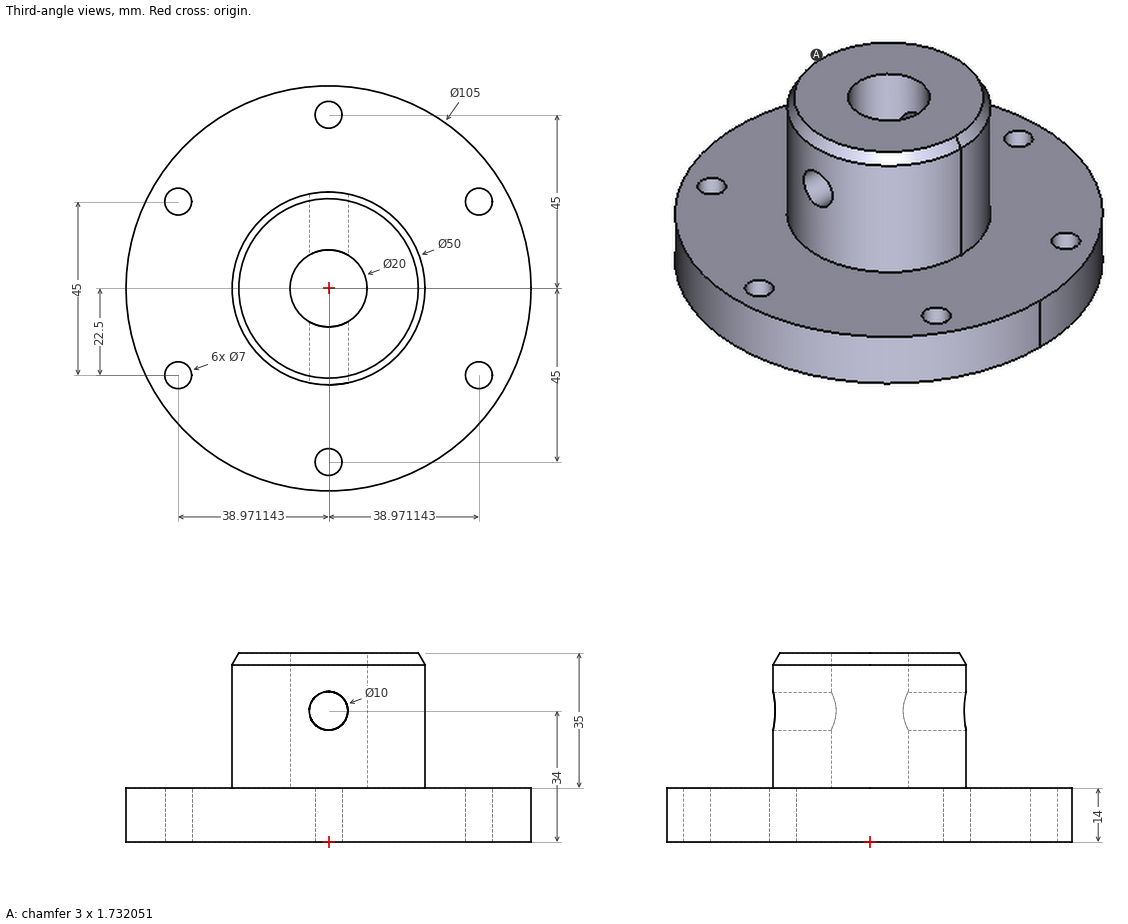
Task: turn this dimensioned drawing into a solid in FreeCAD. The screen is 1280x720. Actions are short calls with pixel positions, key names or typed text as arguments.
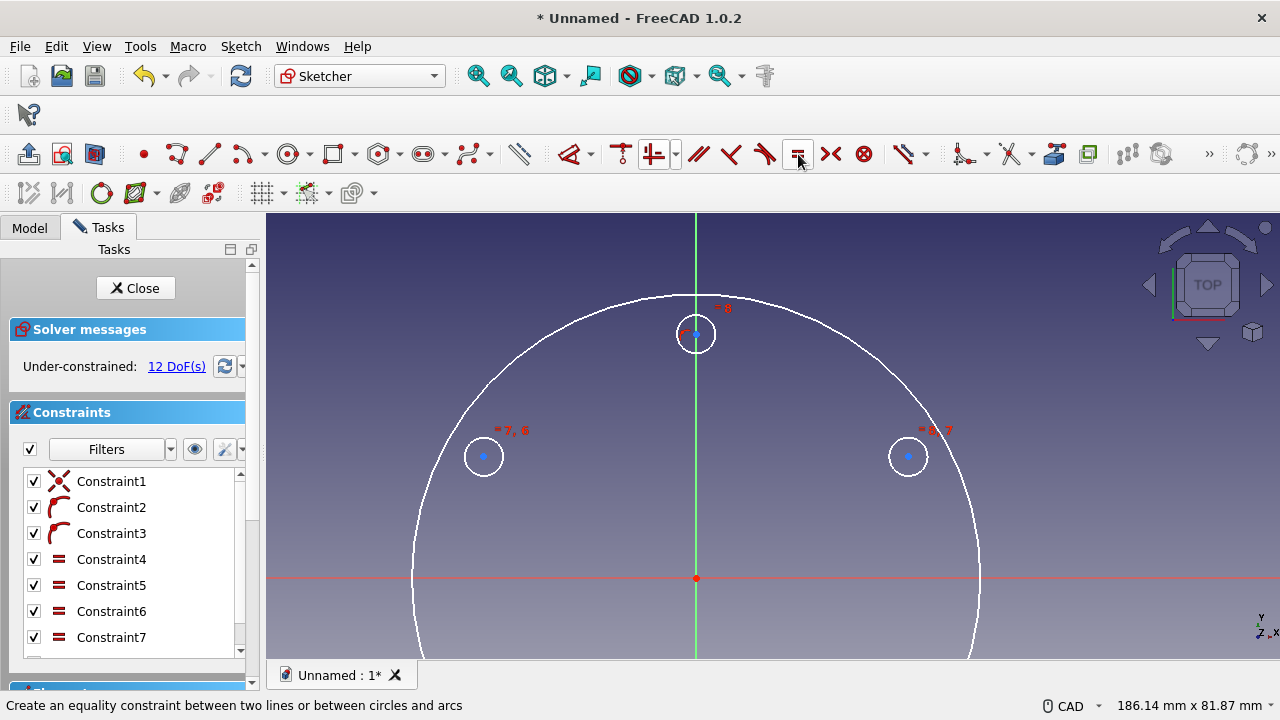
scroll(711, 320, down, 4)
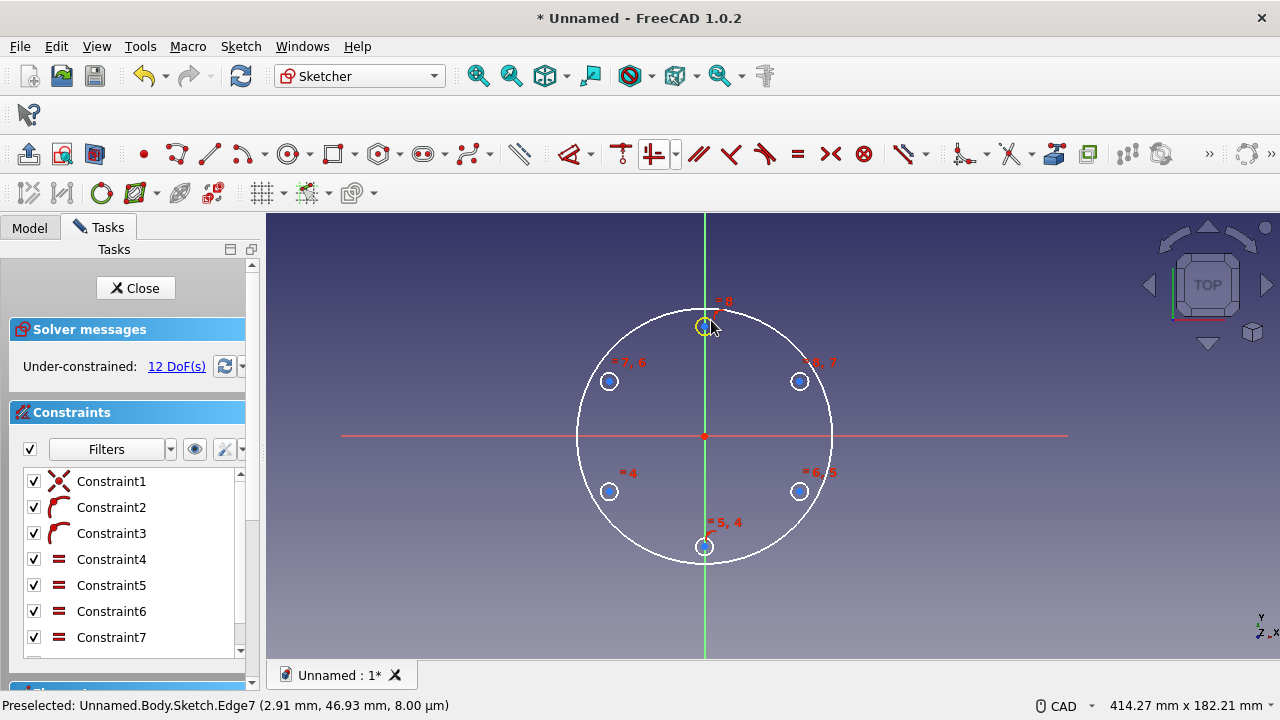
click(609, 492)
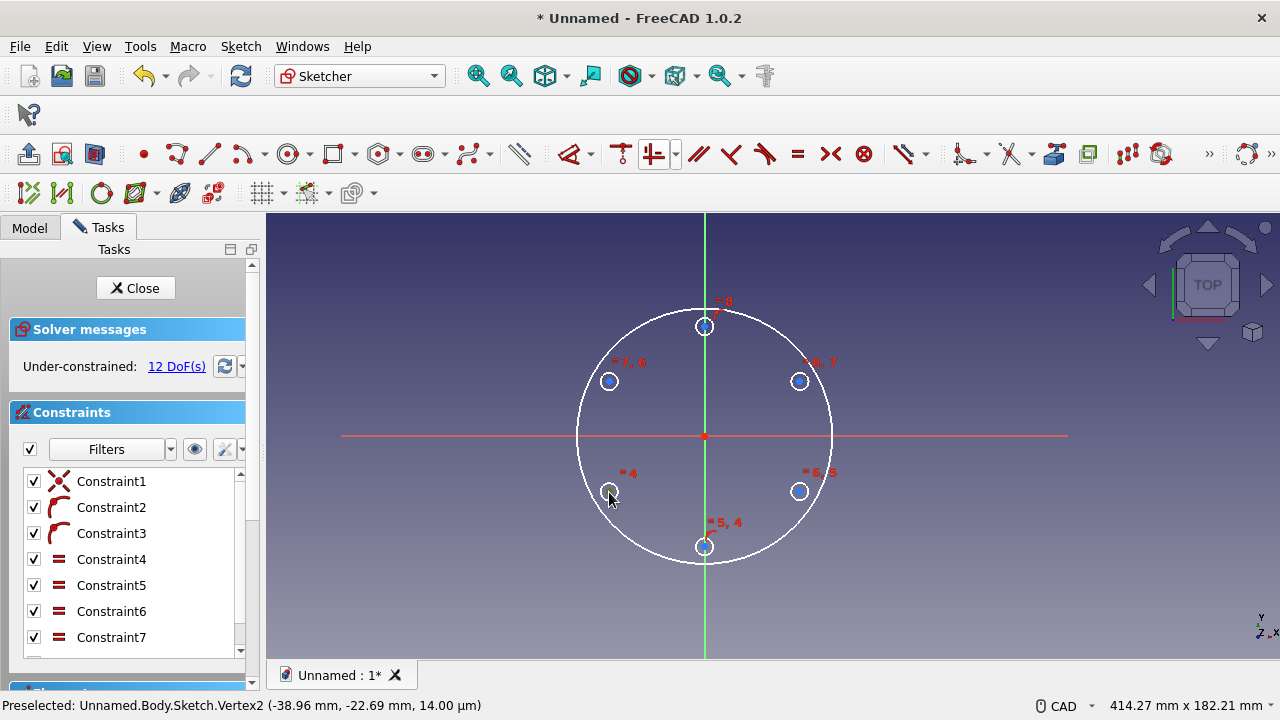
click(800, 492)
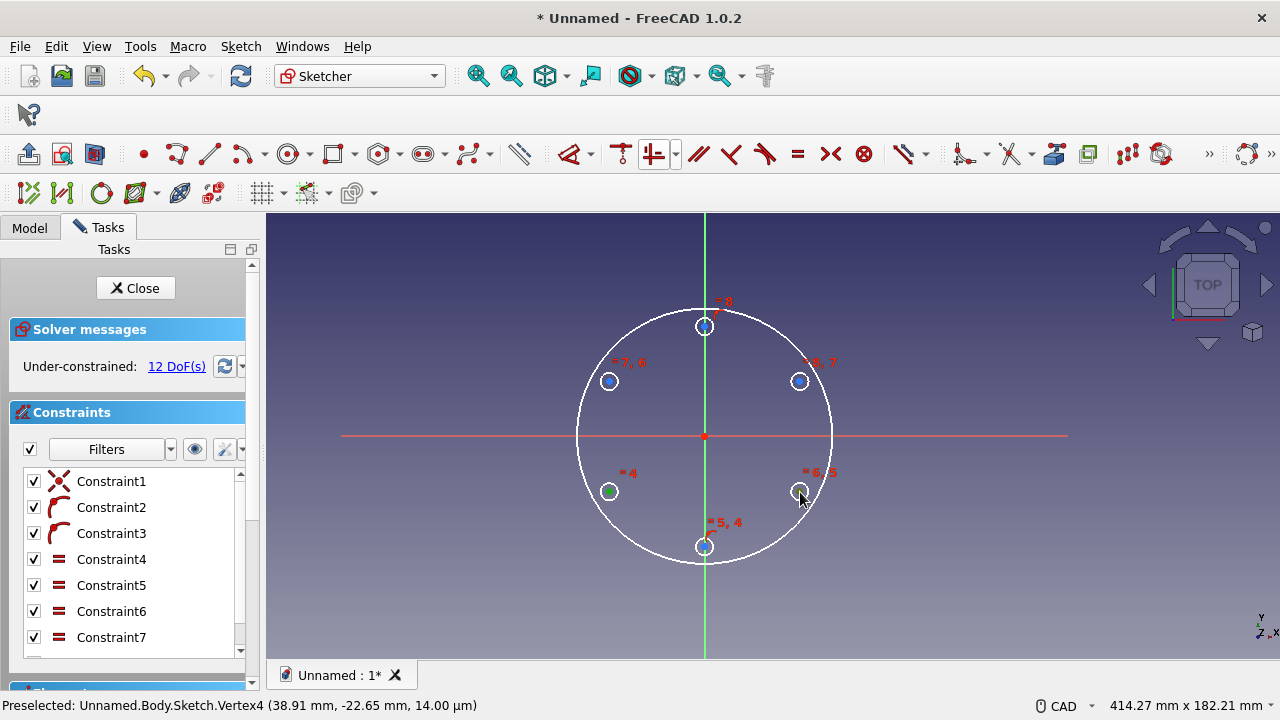
click(676, 154)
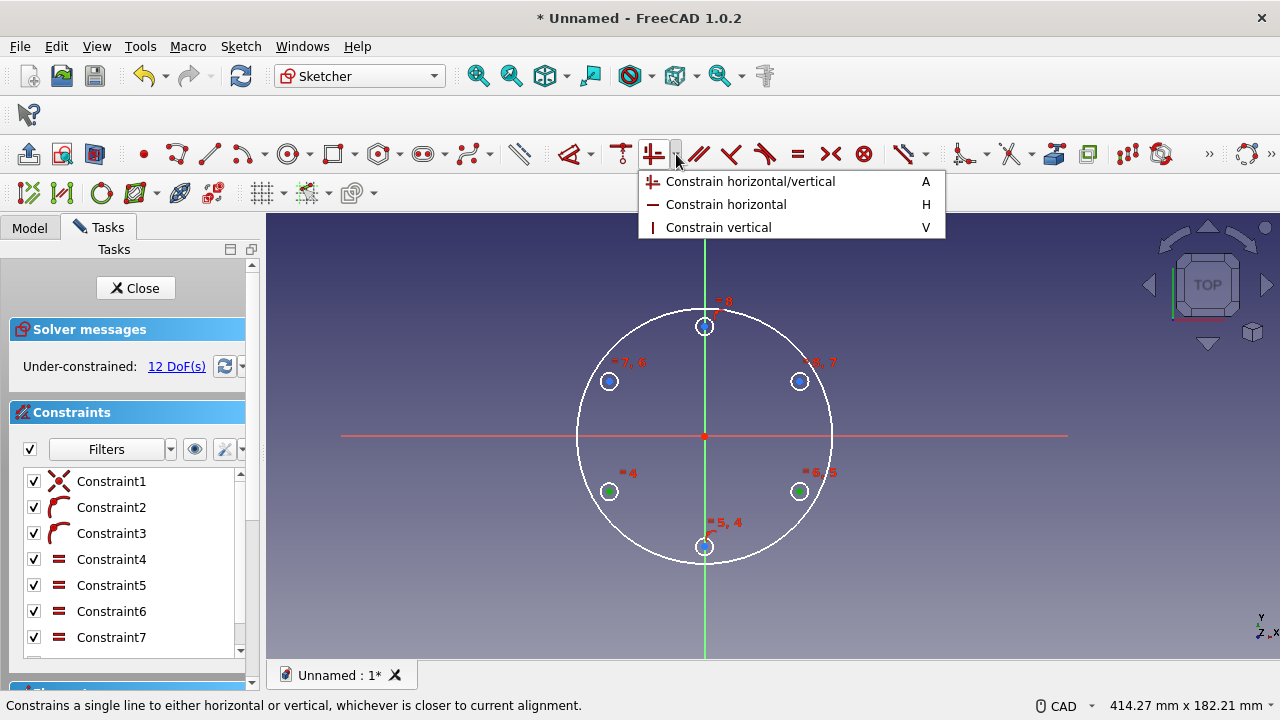
click(792, 204)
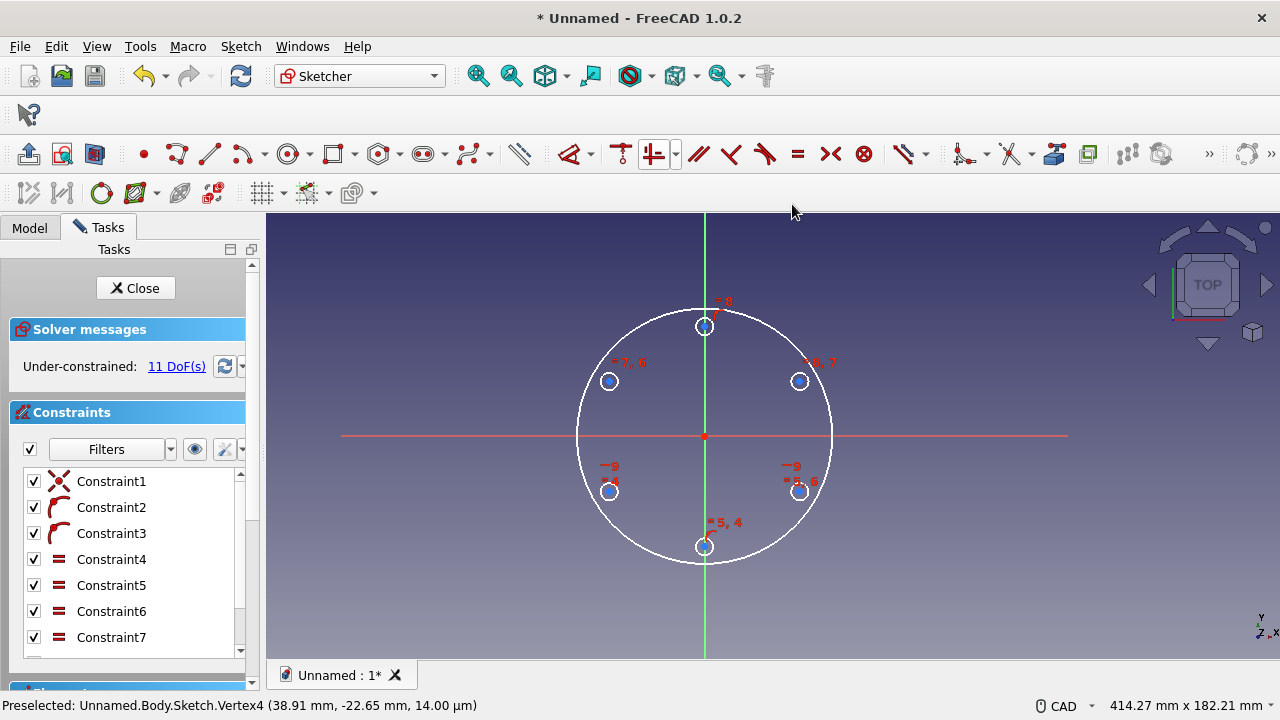
click(609, 492)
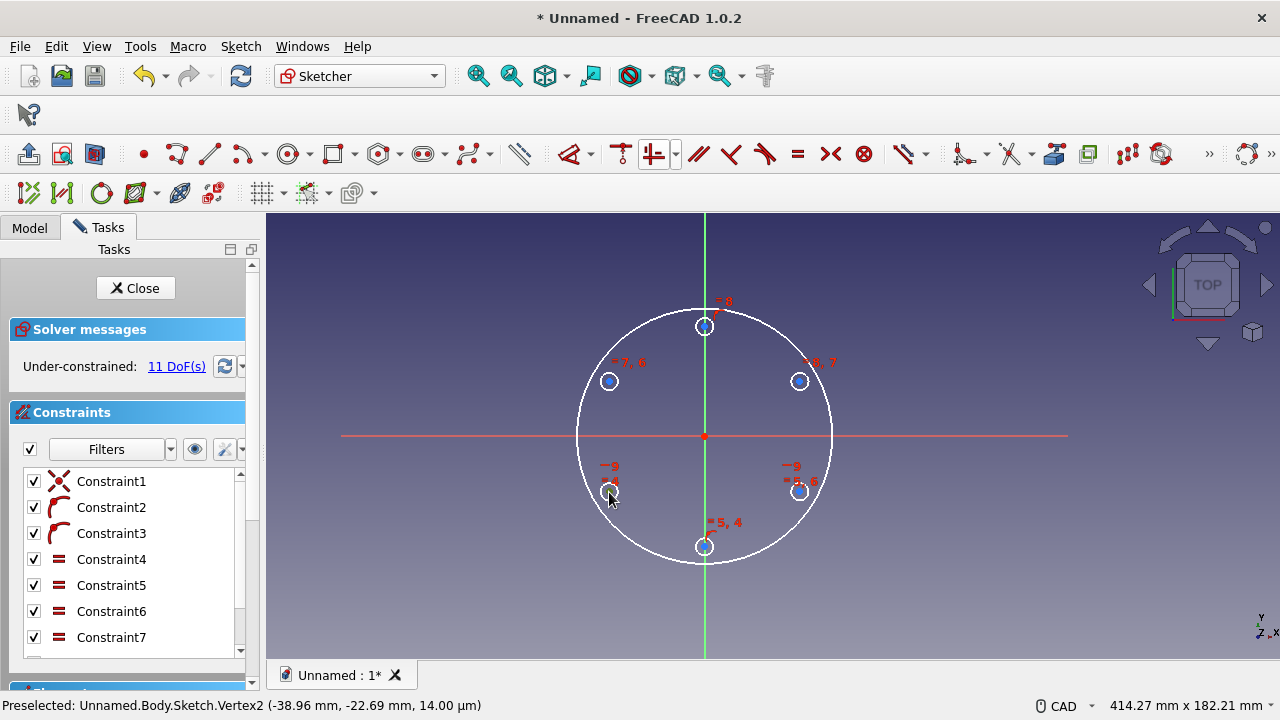
click(609, 382)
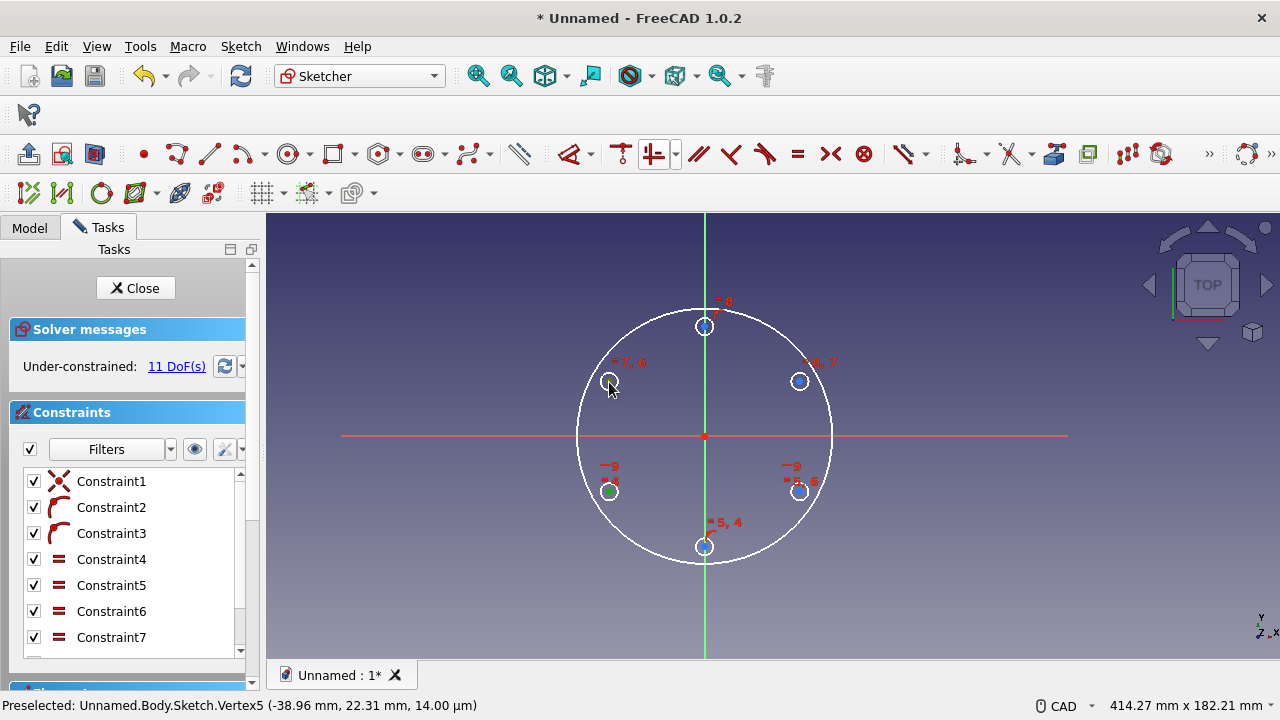
click(676, 154)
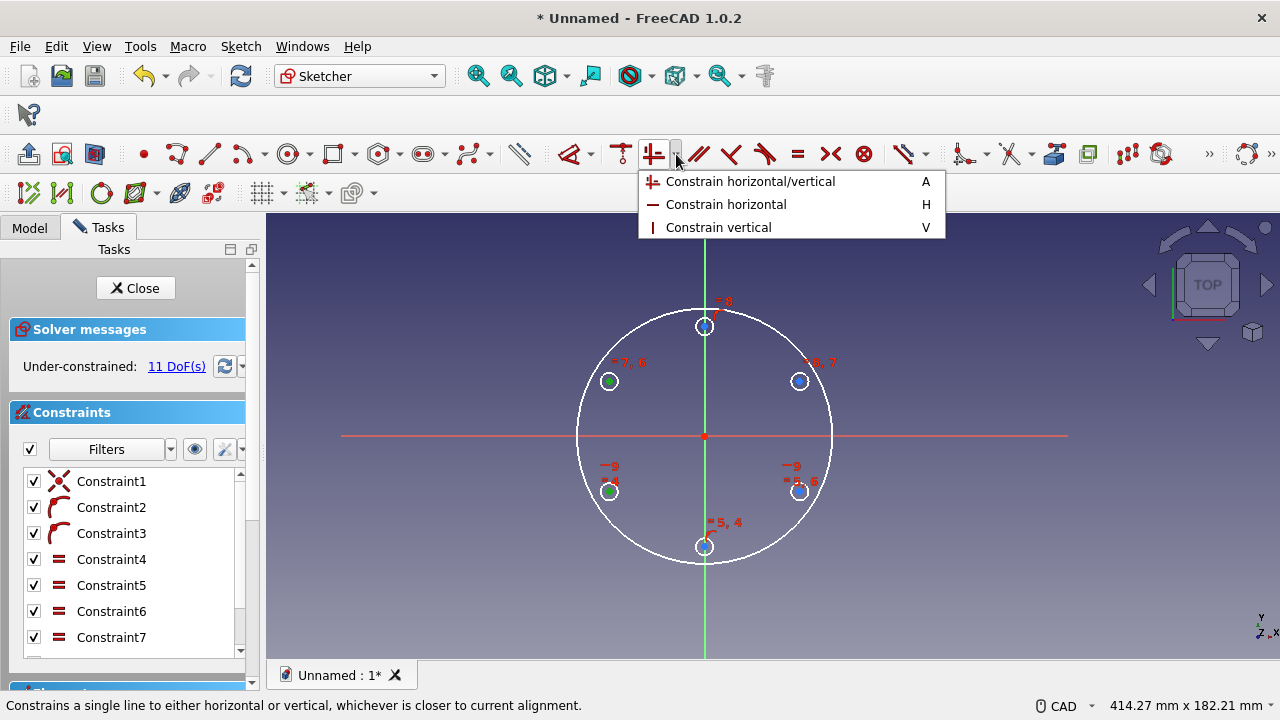
click(792, 228)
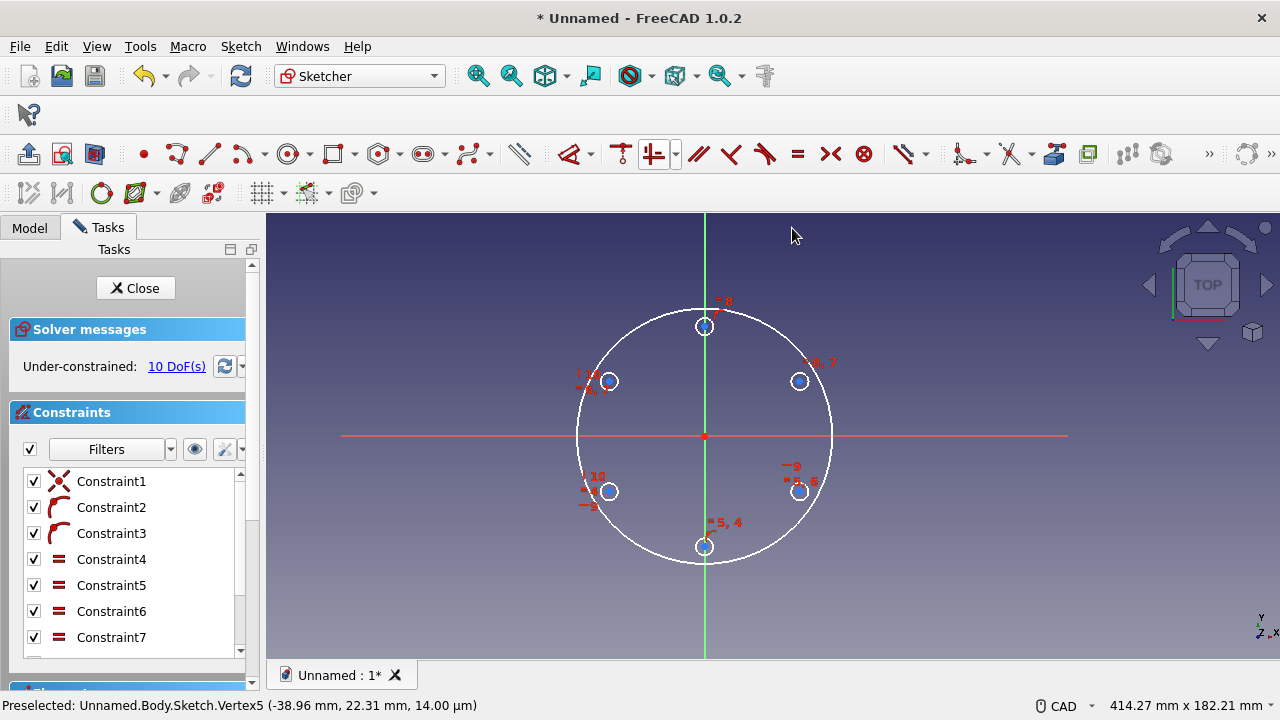
click(800, 492)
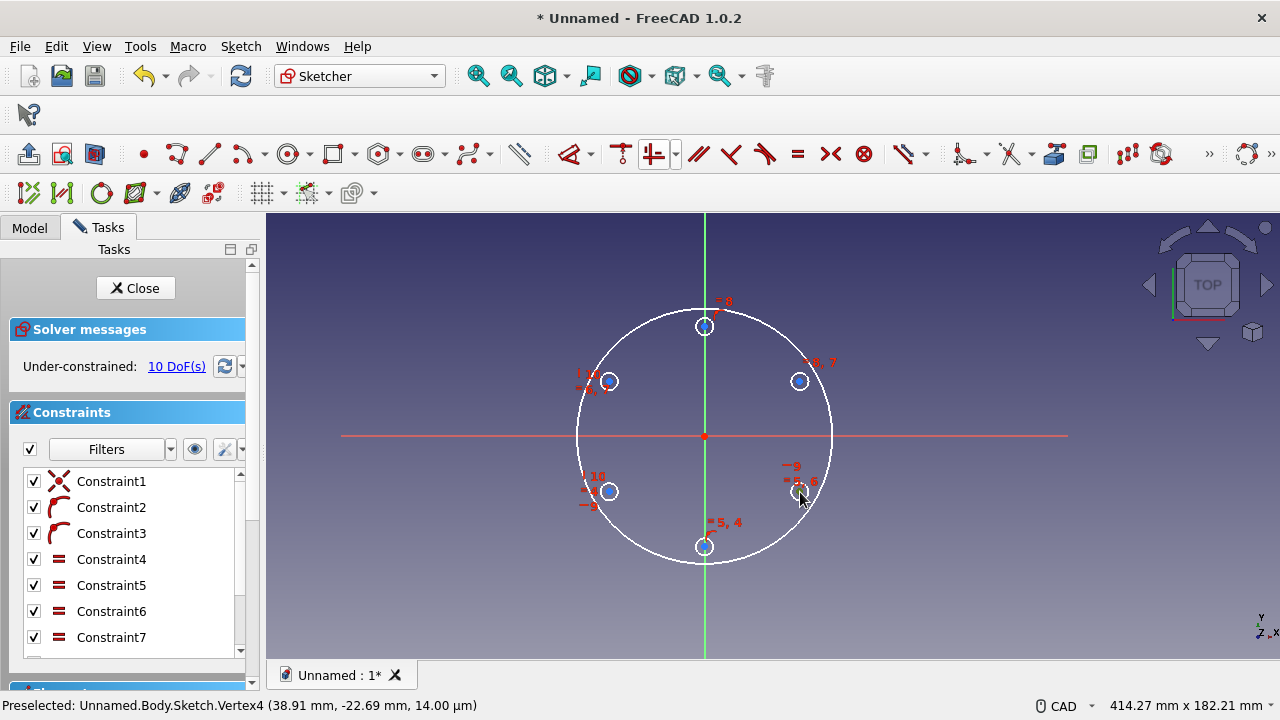
click(800, 382)